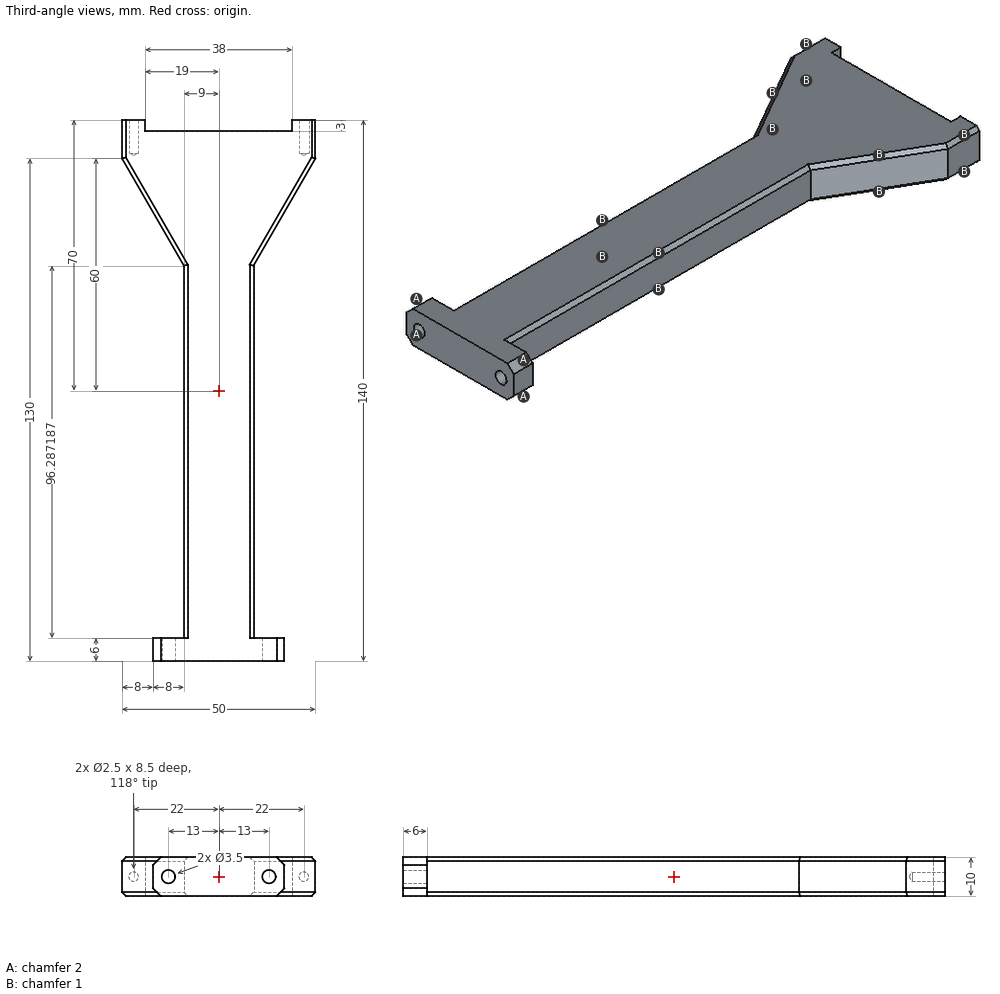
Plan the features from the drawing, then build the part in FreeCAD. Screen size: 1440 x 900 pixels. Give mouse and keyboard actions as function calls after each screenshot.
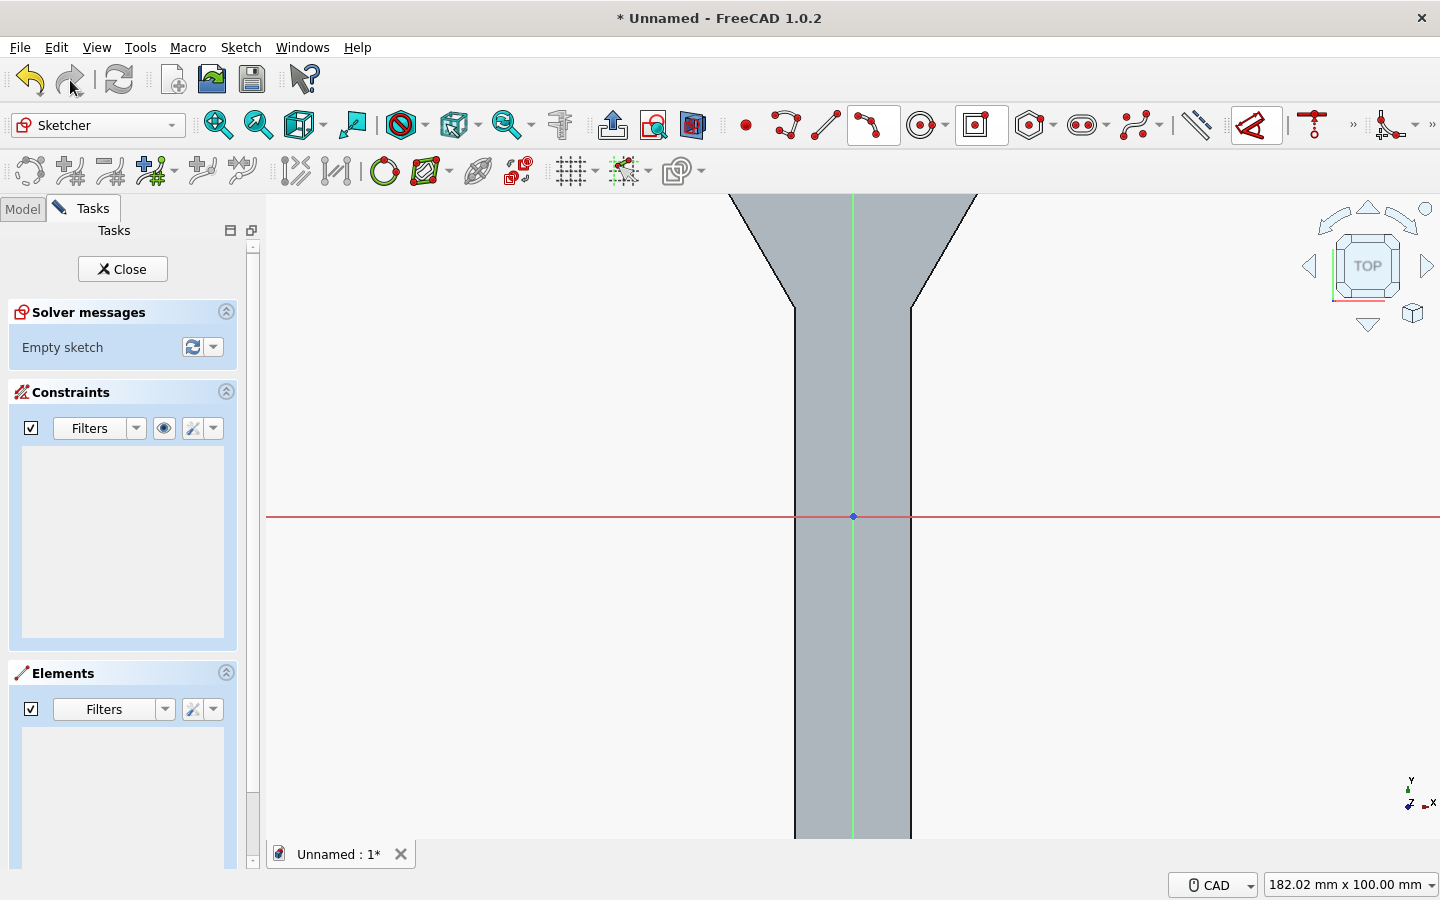
scroll(645, 811, down, 2)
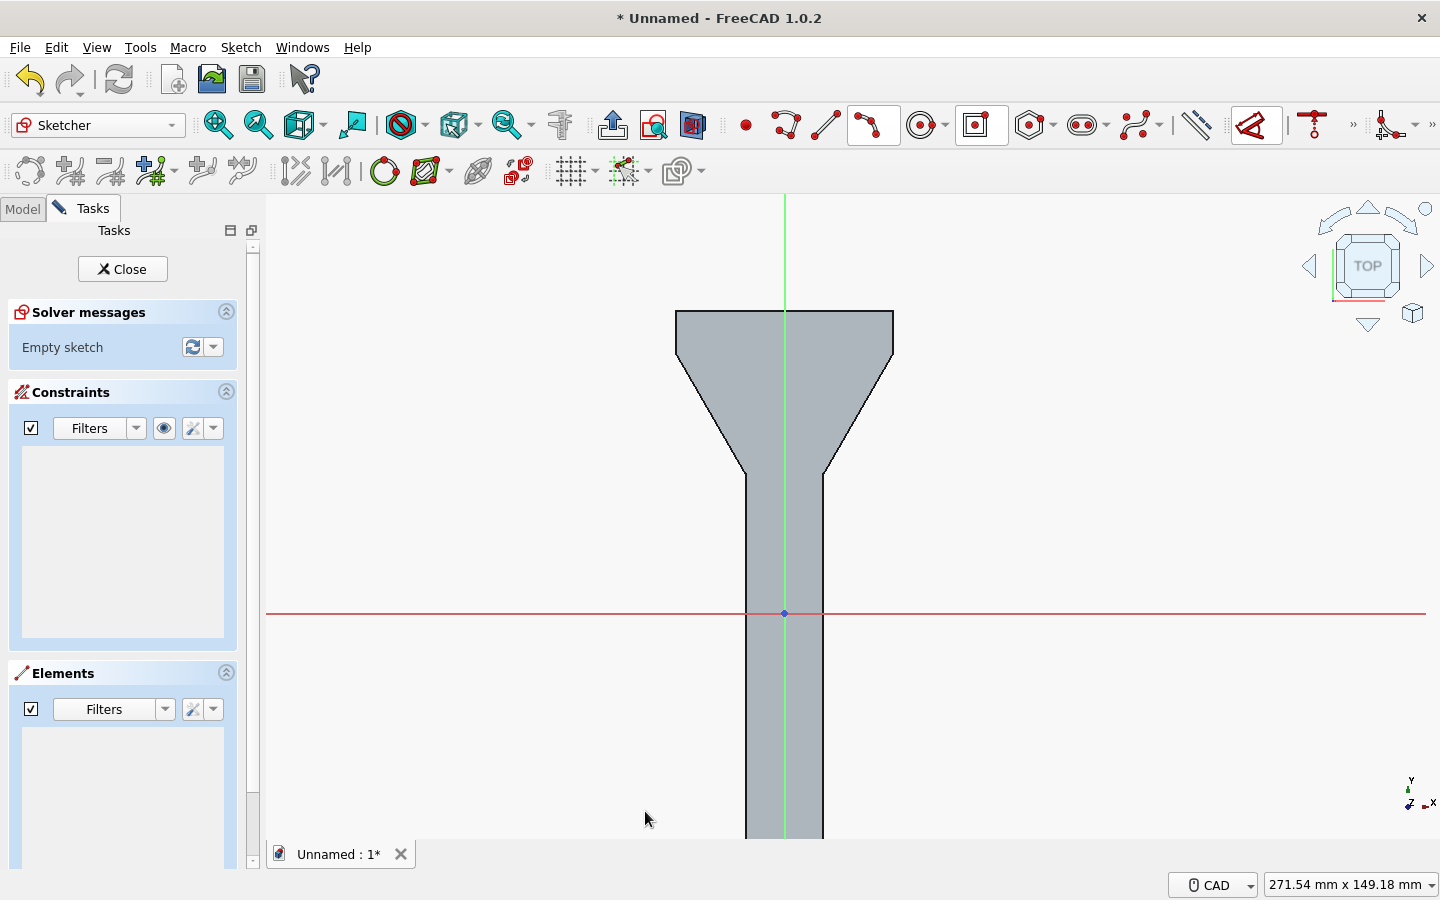
scroll(785, 353, up, 2)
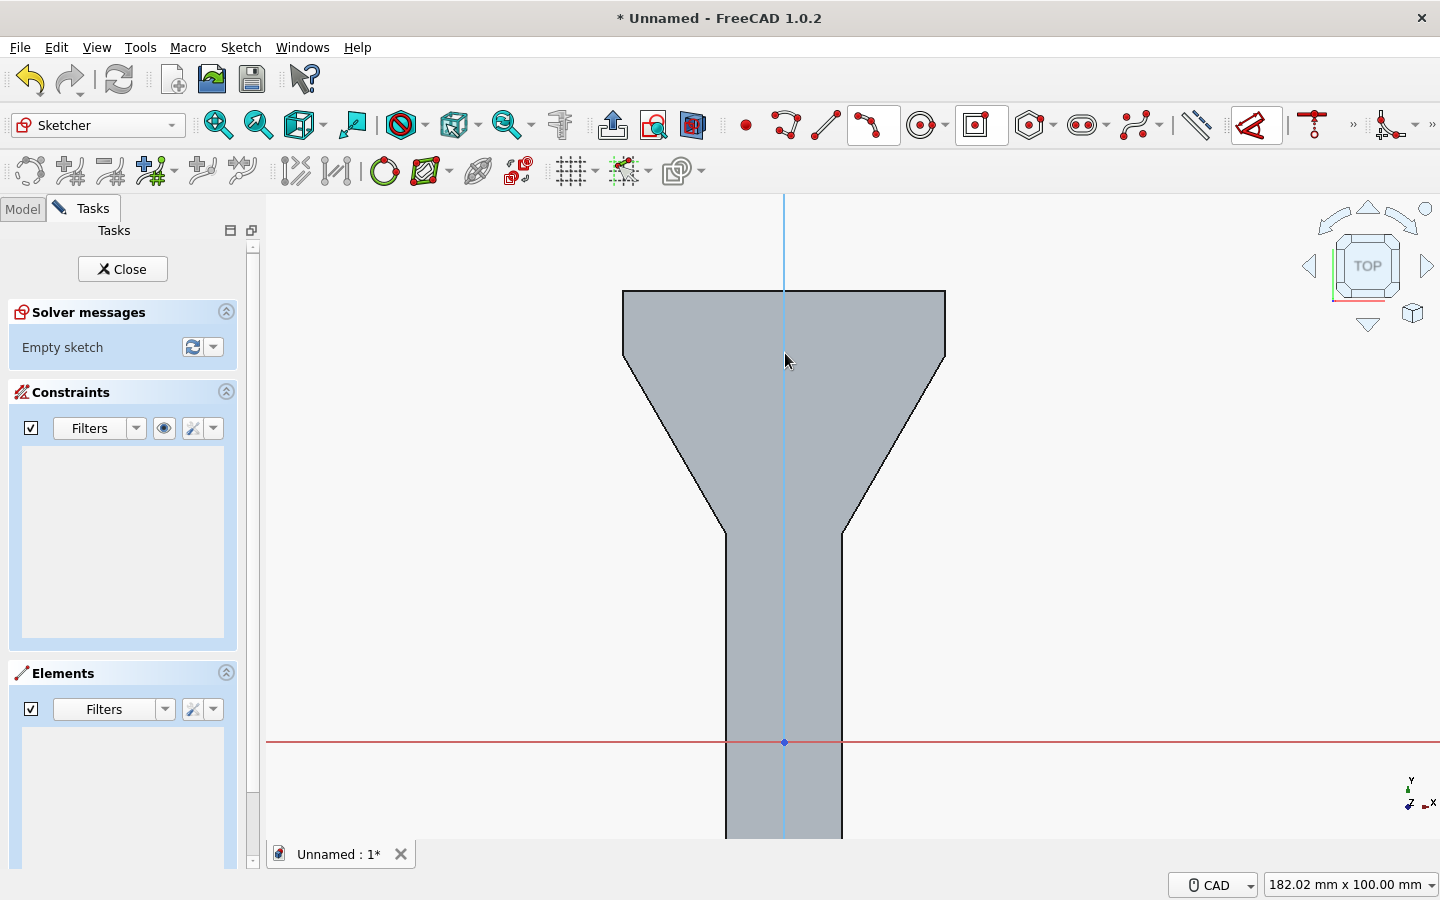
click(1002, 126)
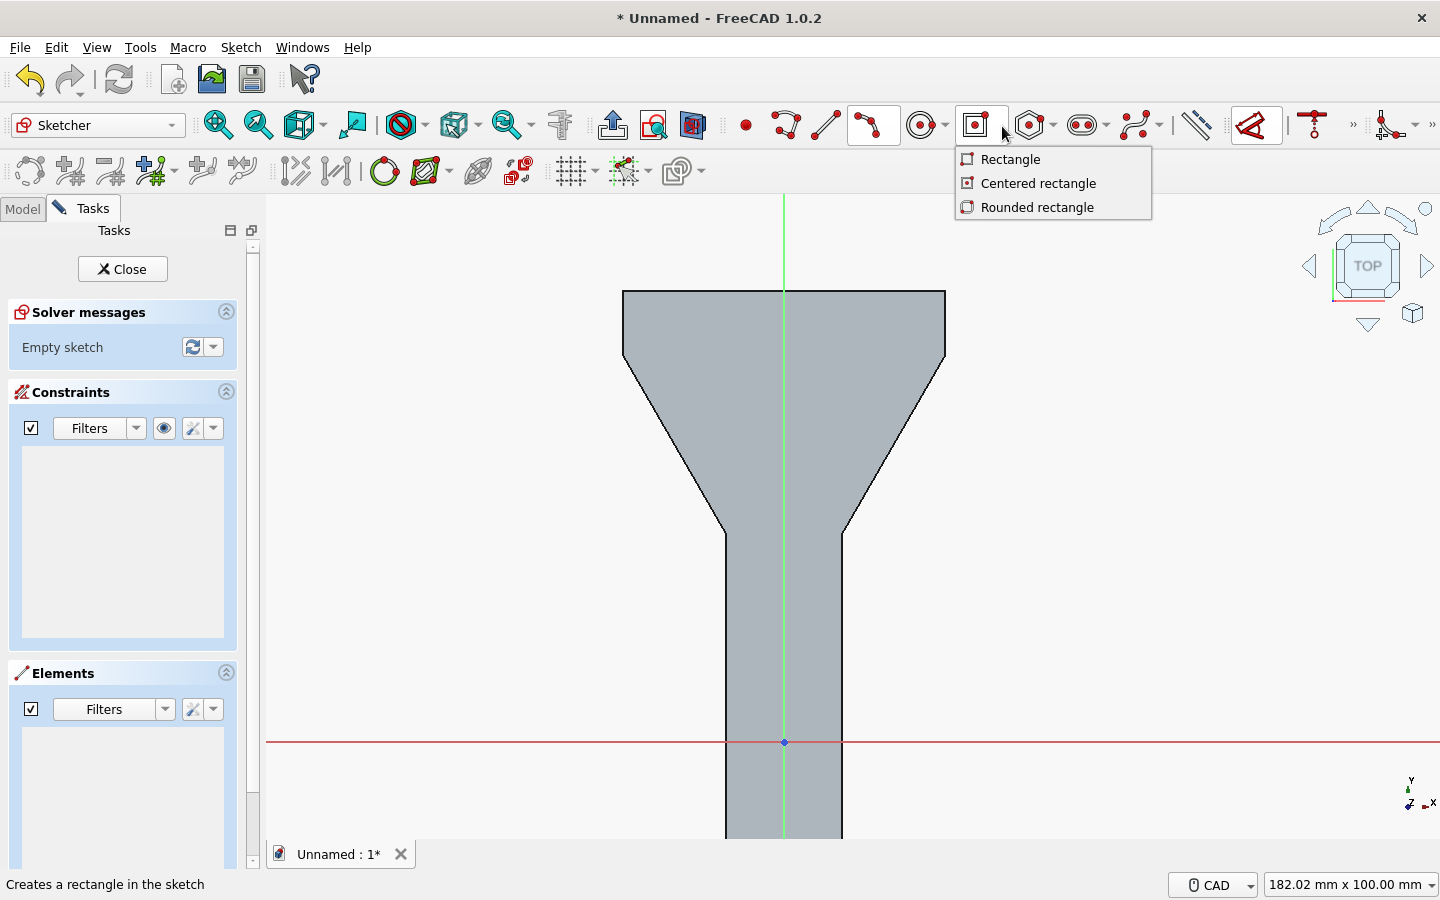
click(1054, 159)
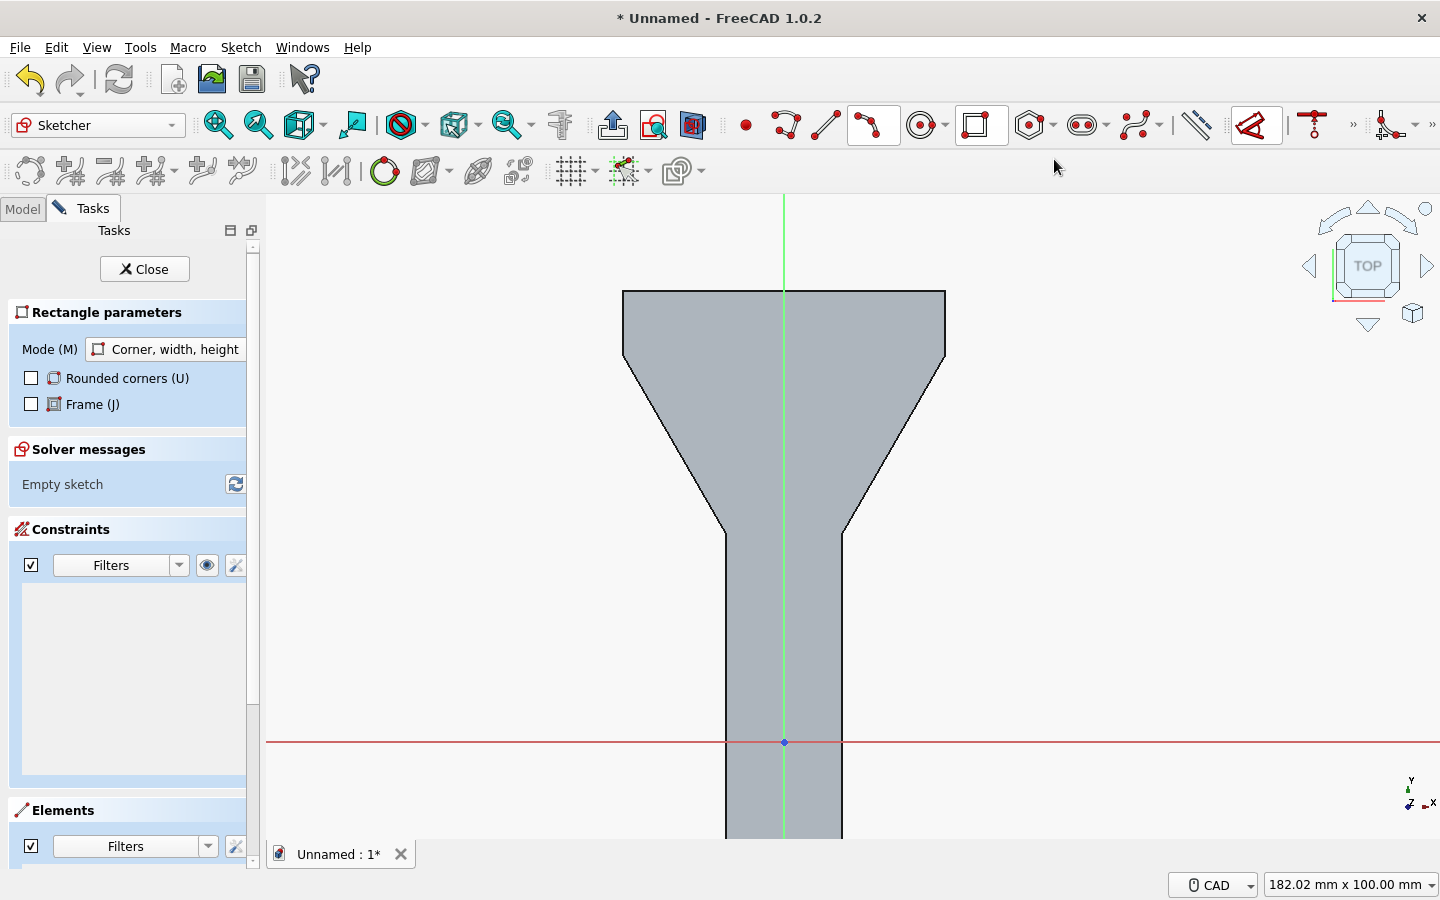
click(662, 291)
move(907, 310)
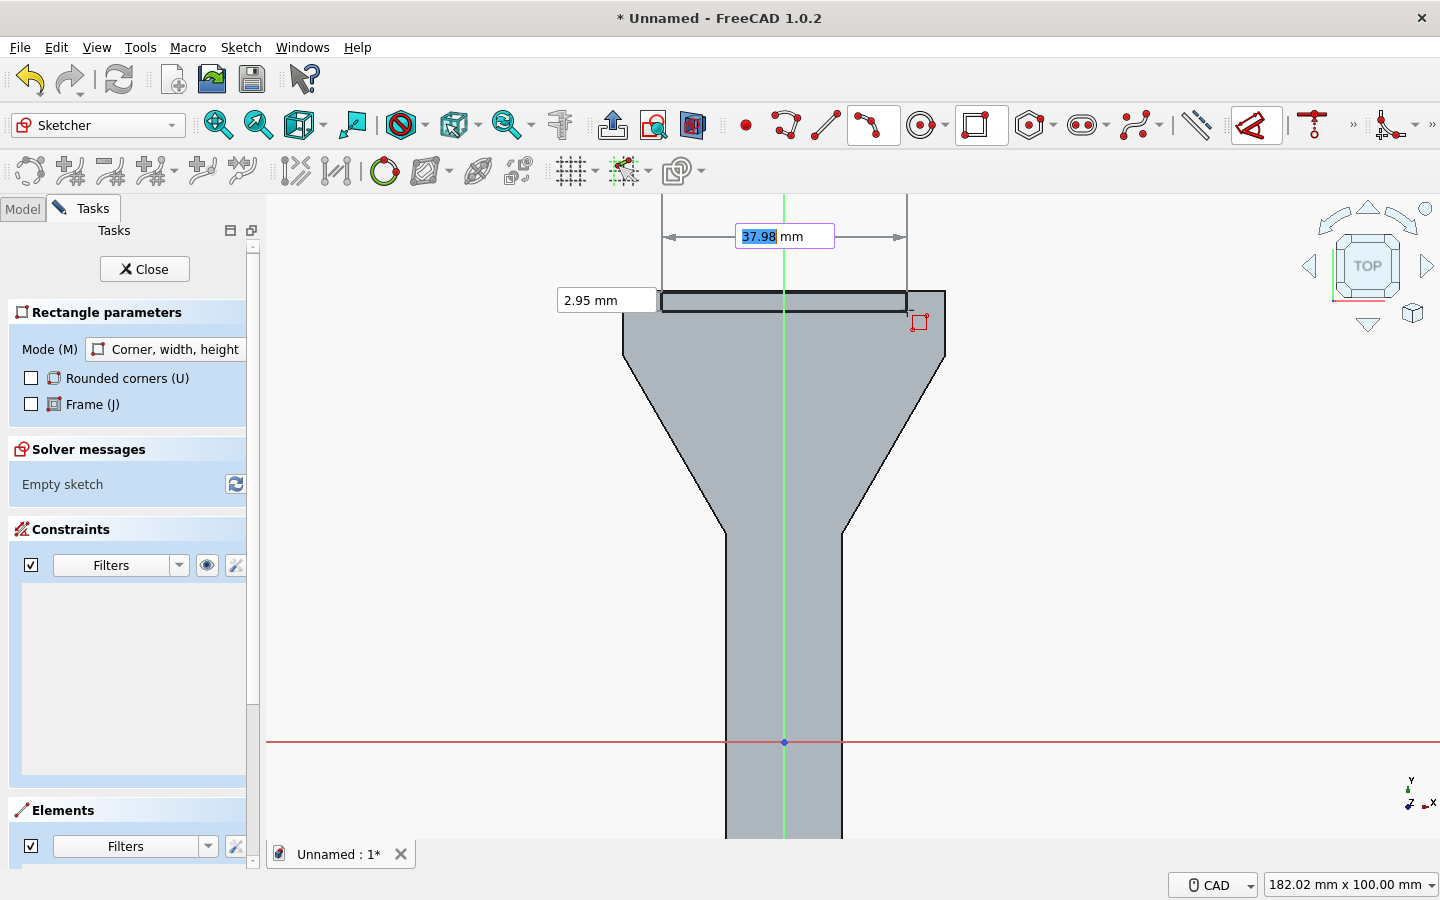
text(38)
key(Tab)
text(3)
key(Return)
key(Escape)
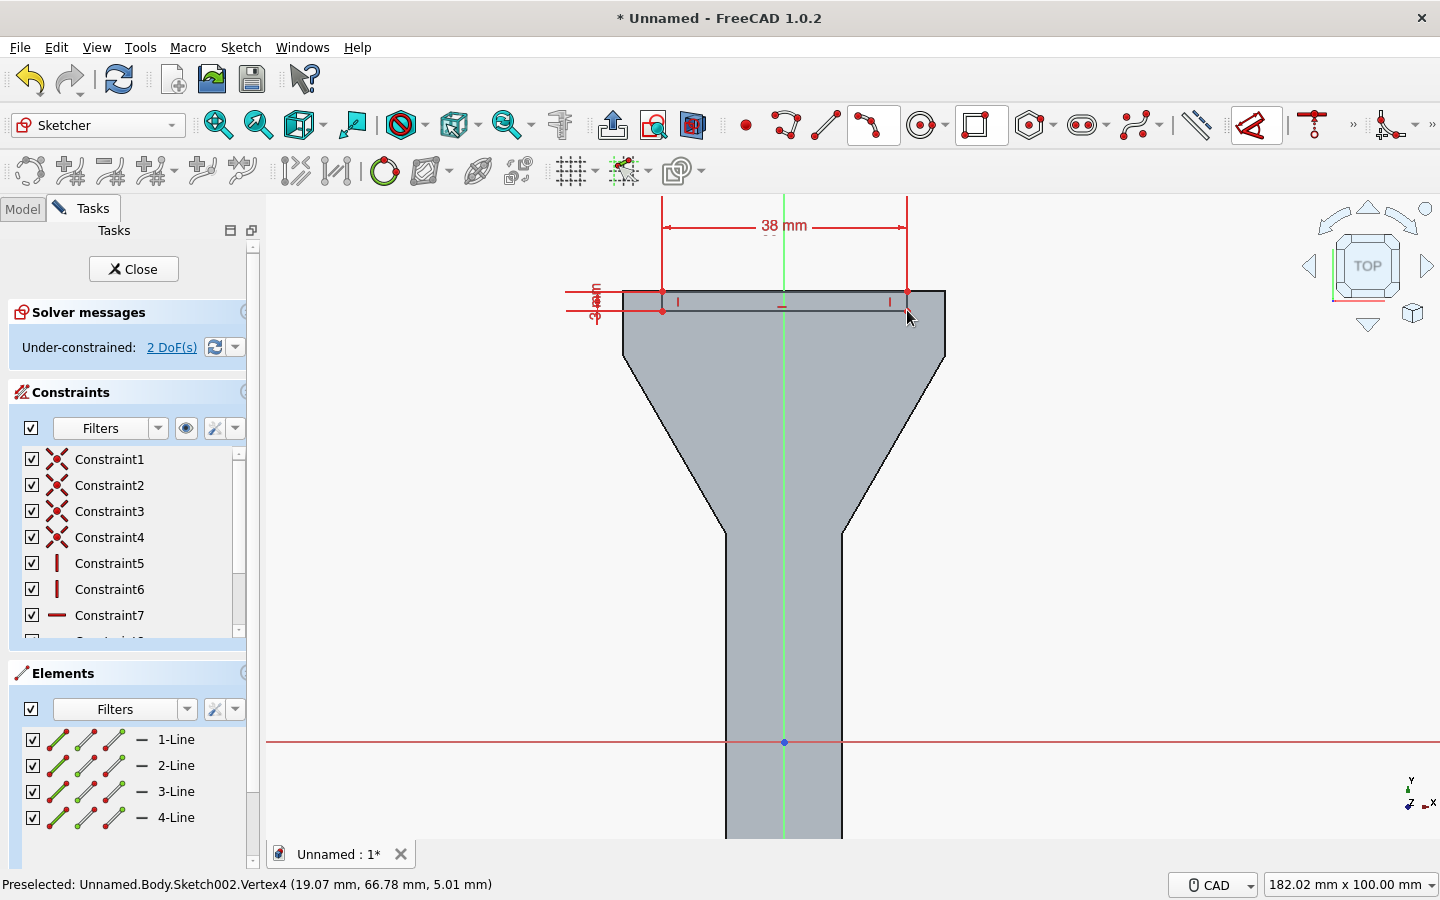
click(662, 292)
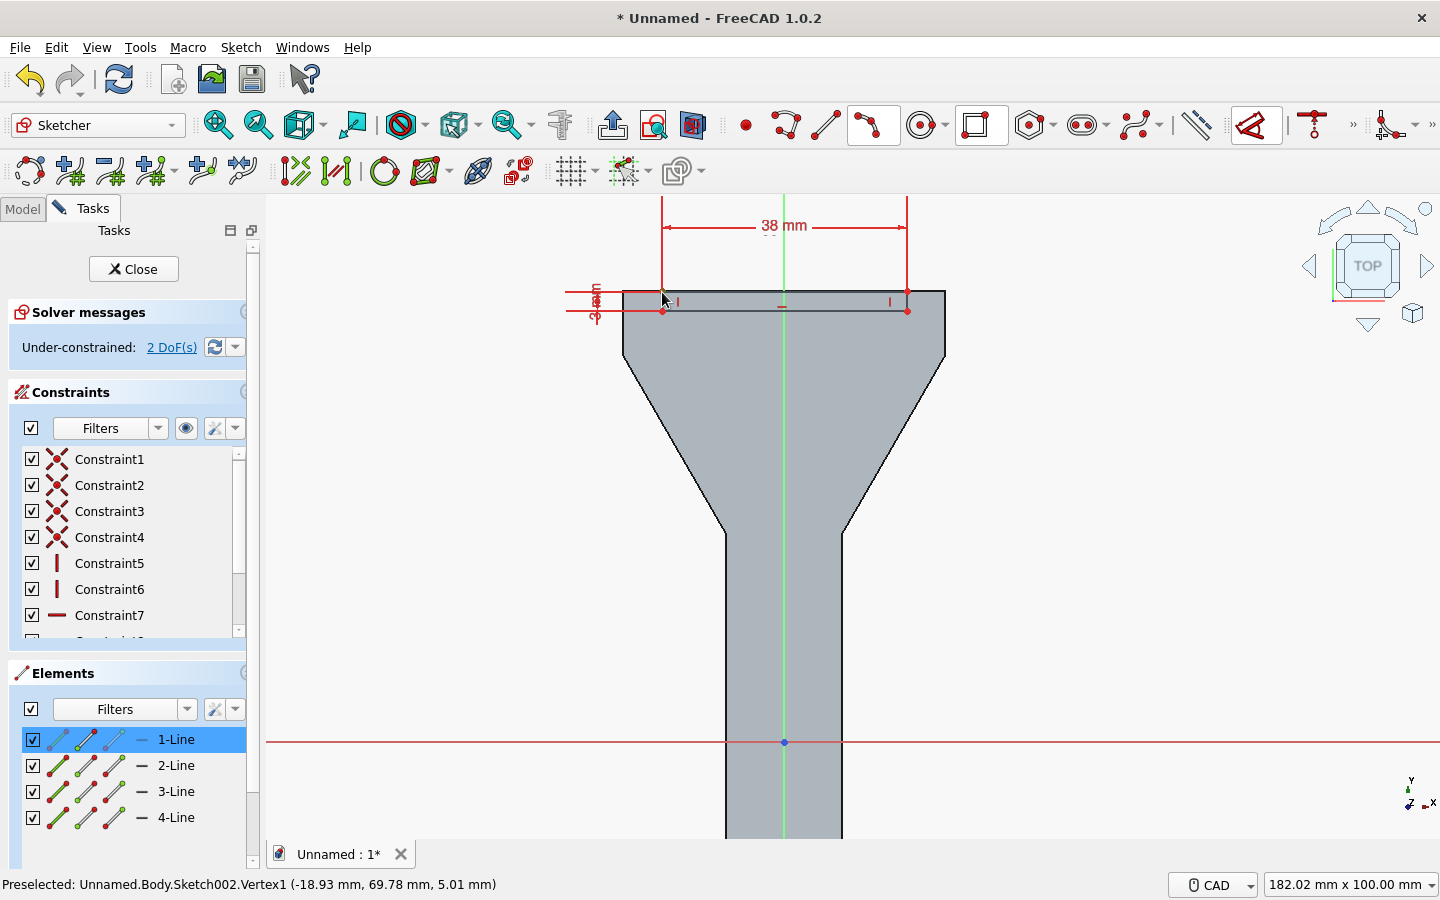
click(1276, 126)